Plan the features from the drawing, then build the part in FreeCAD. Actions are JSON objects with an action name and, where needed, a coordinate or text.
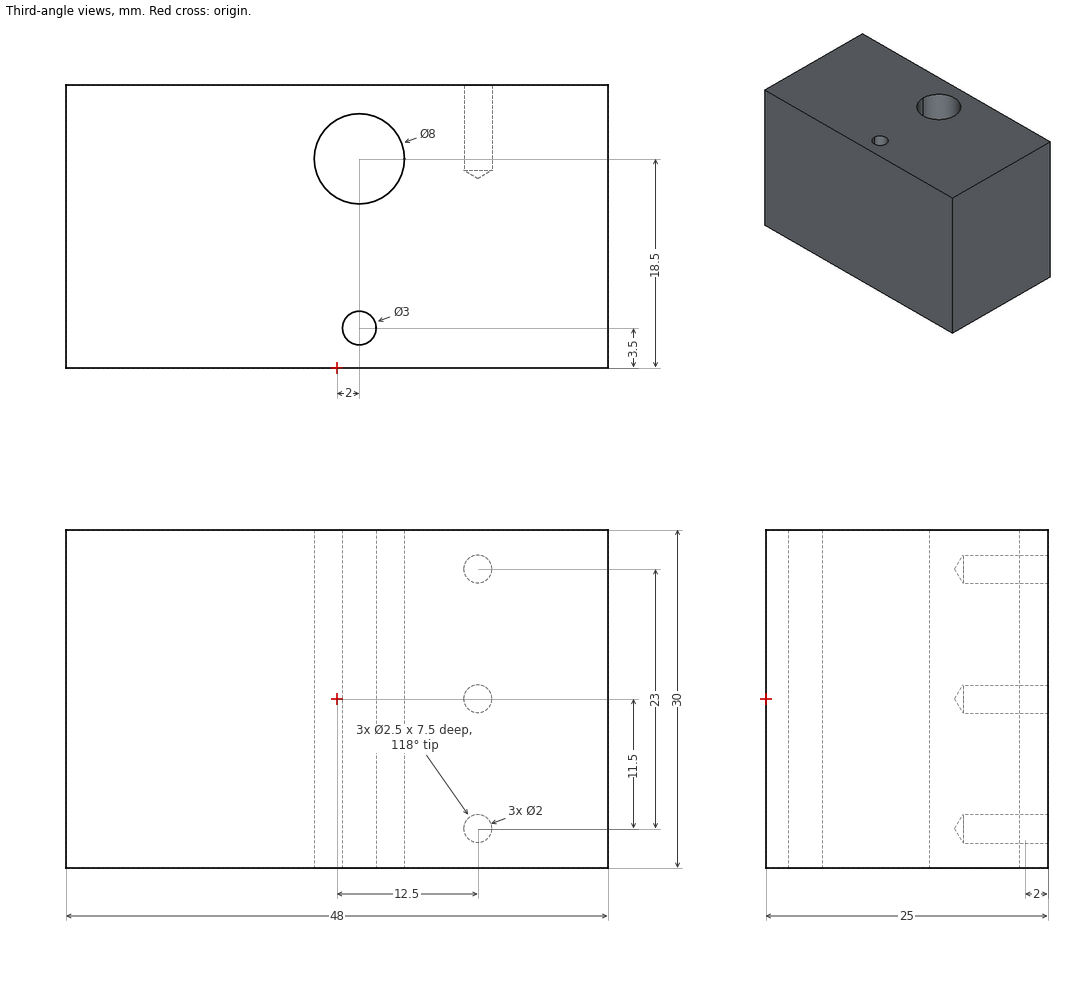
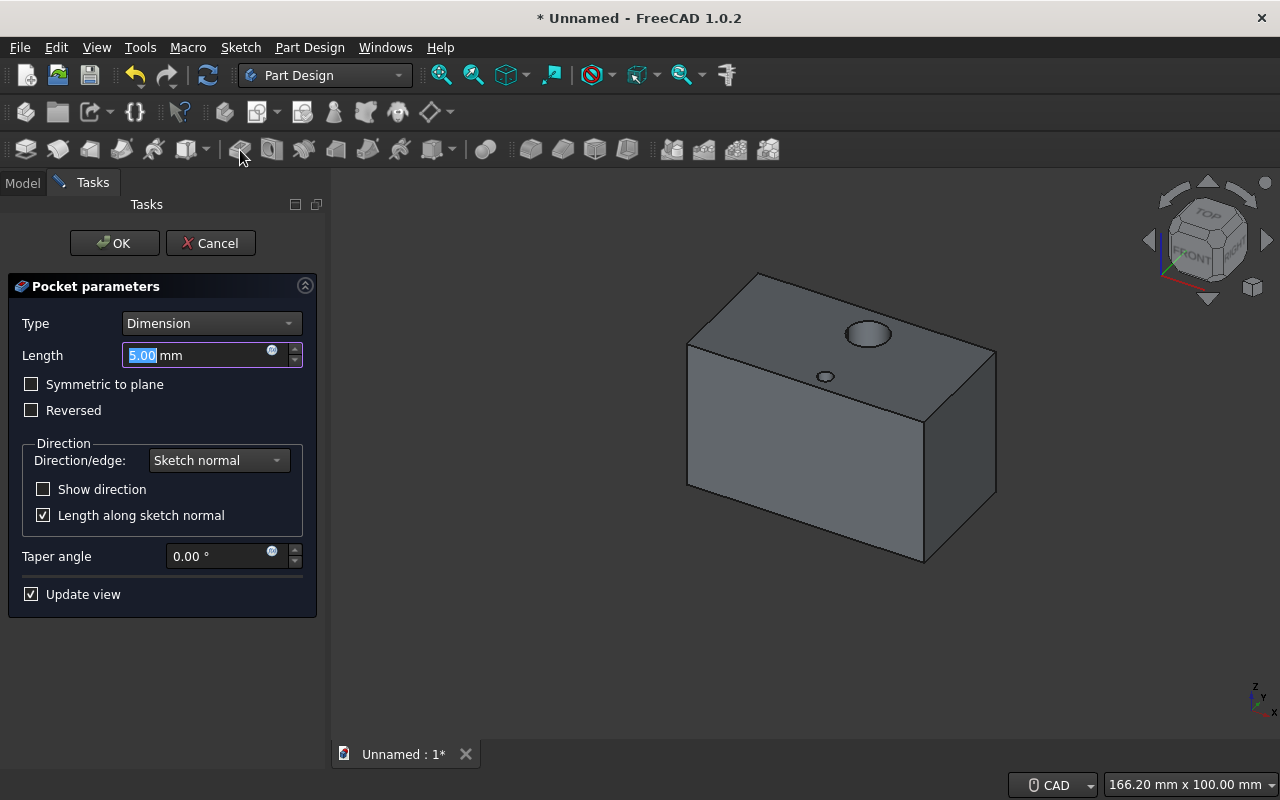
{"action": "left_click", "coordinate": [212, 324]}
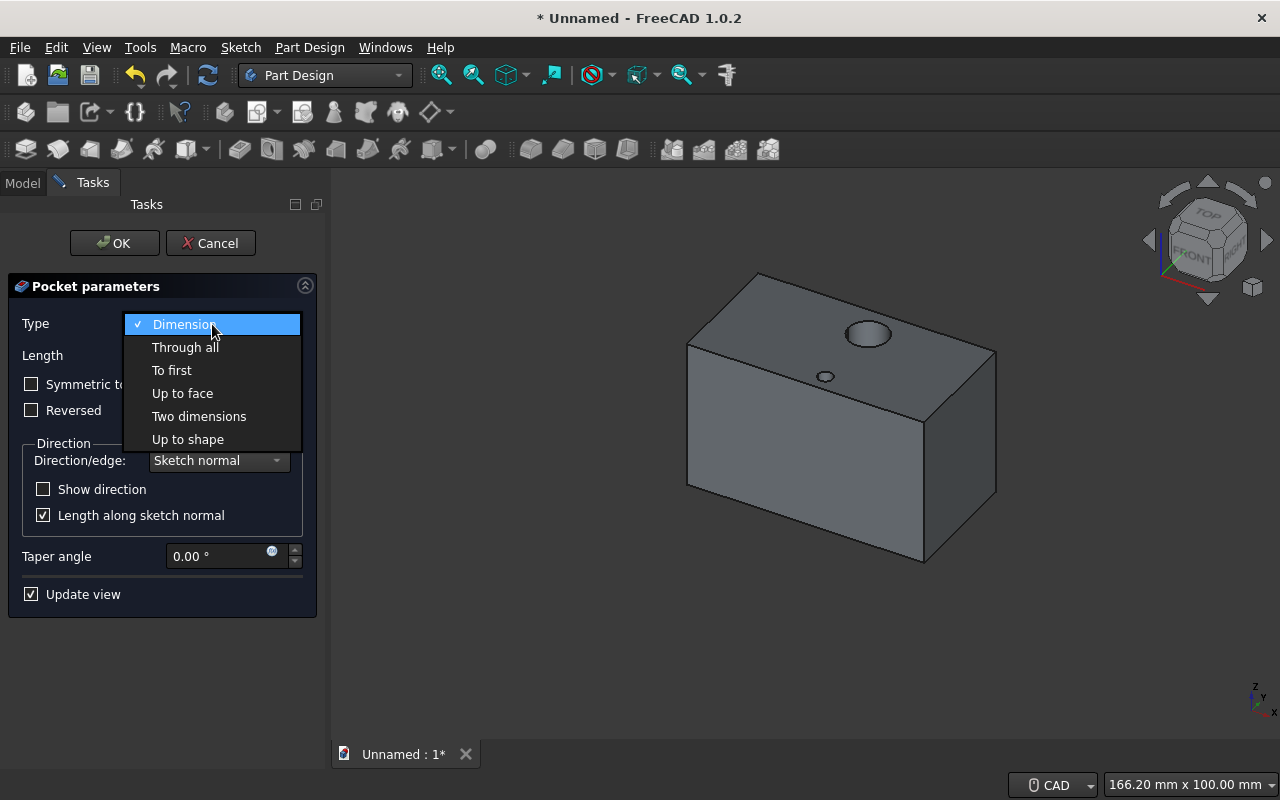
{"action": "left_click", "coordinate": [212, 370]}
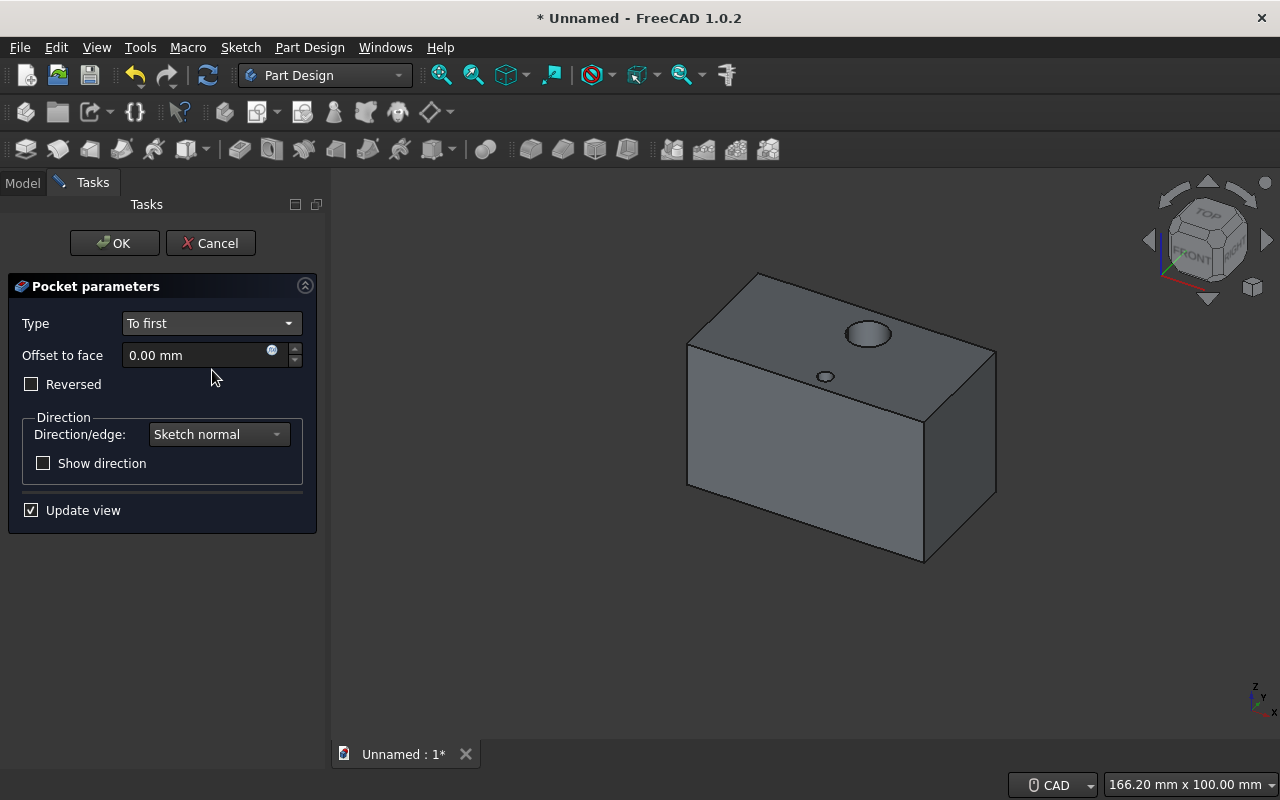
{"action": "left_click", "coordinate": [115, 243]}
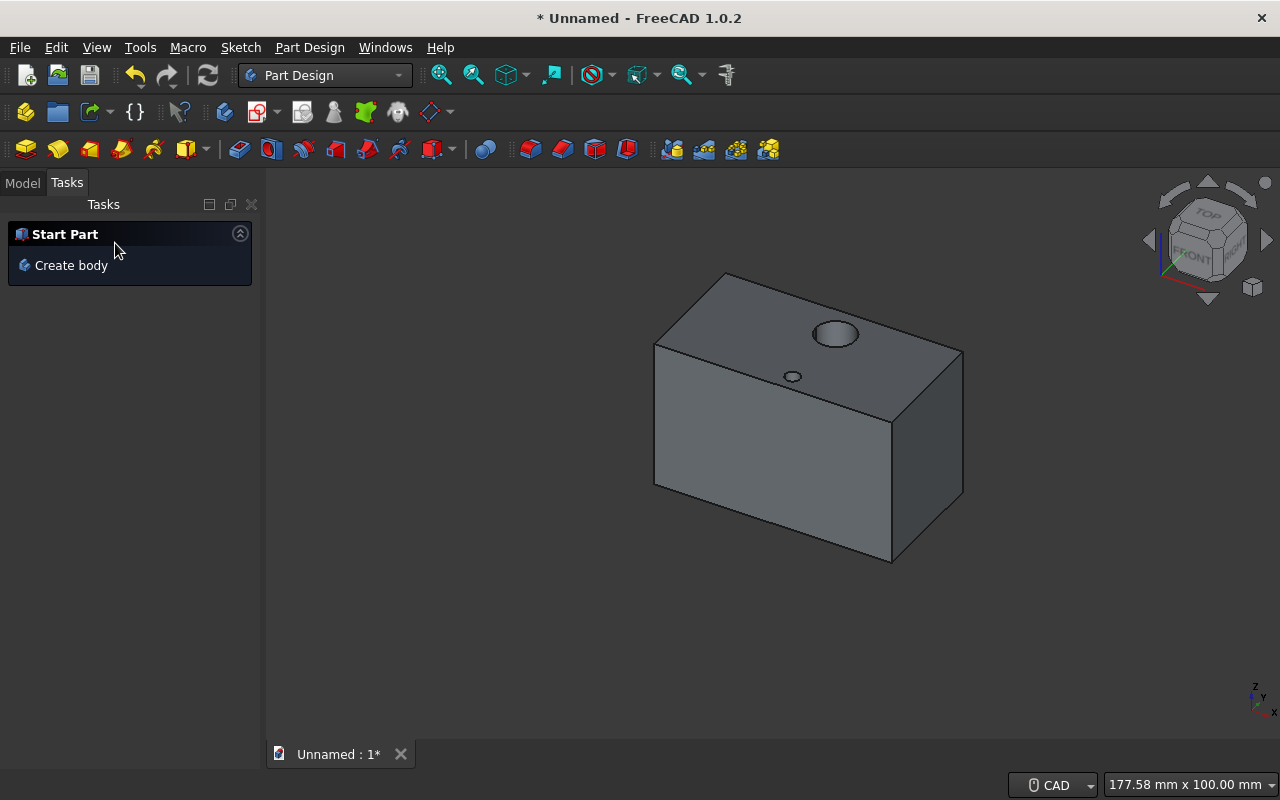
{"action": "key", "text": "4"}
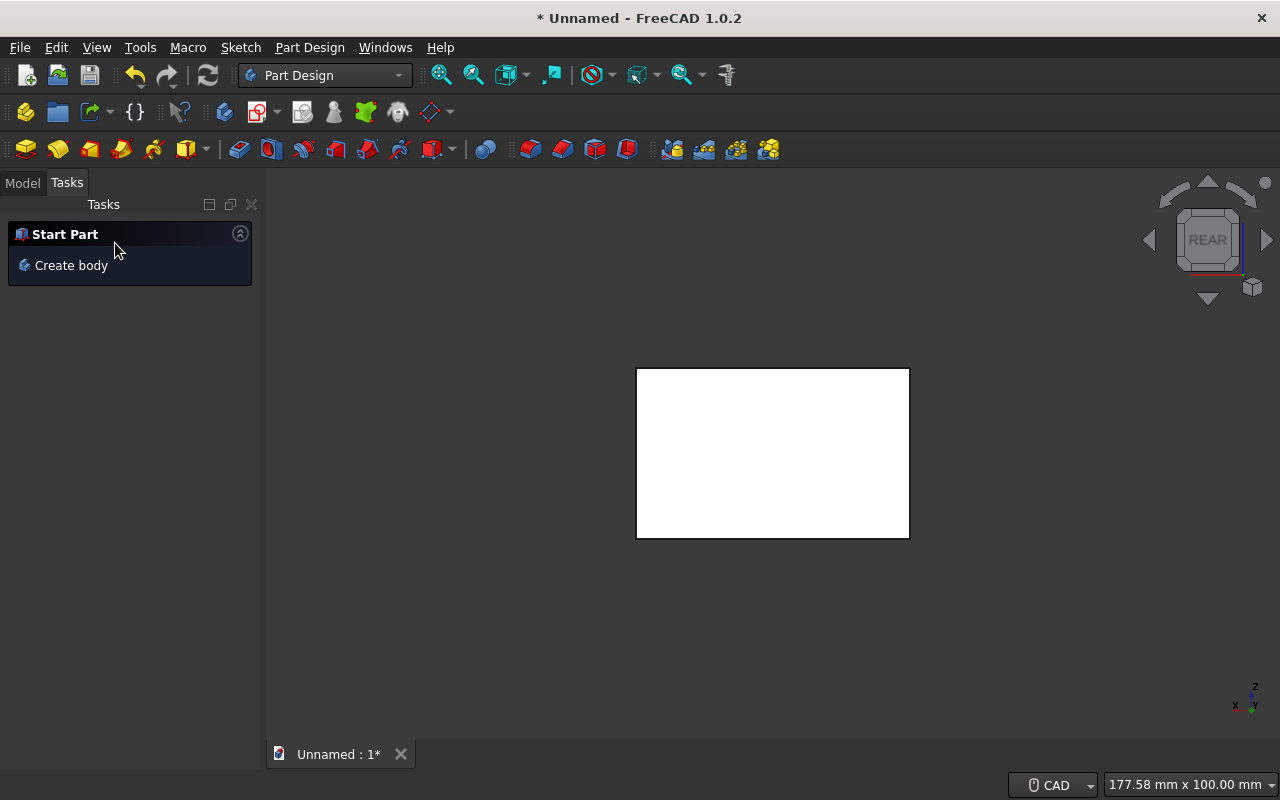
{"action": "key", "text": "v f"}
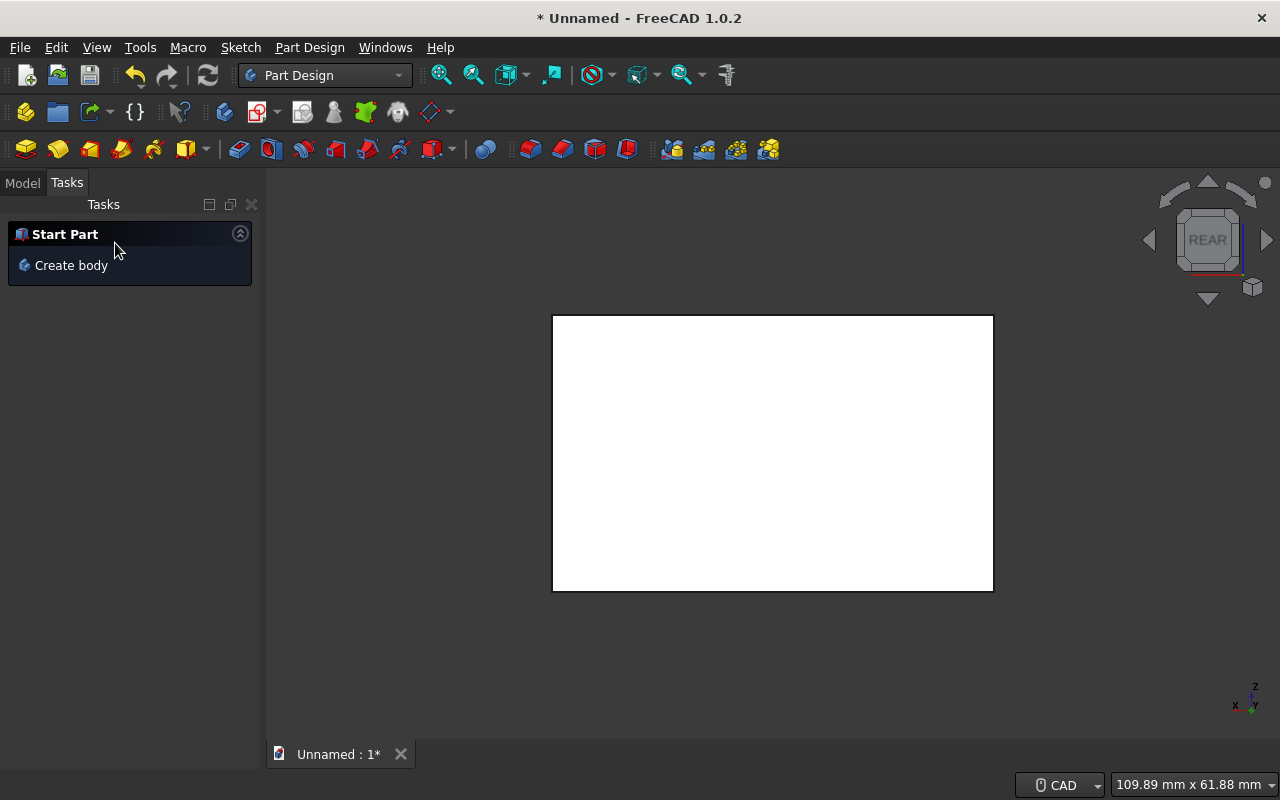
{"action": "left_click", "coordinate": [710, 453]}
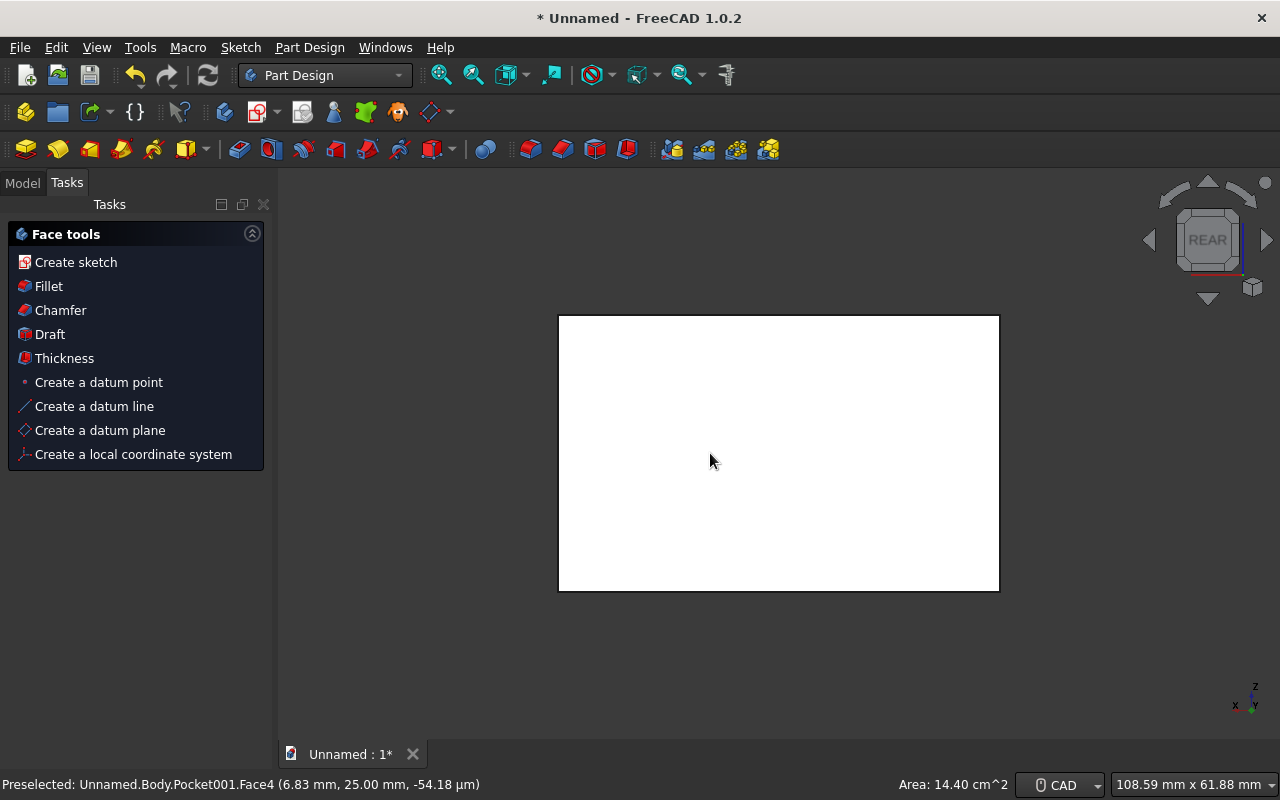
{"action": "left_click", "coordinate": [258, 112]}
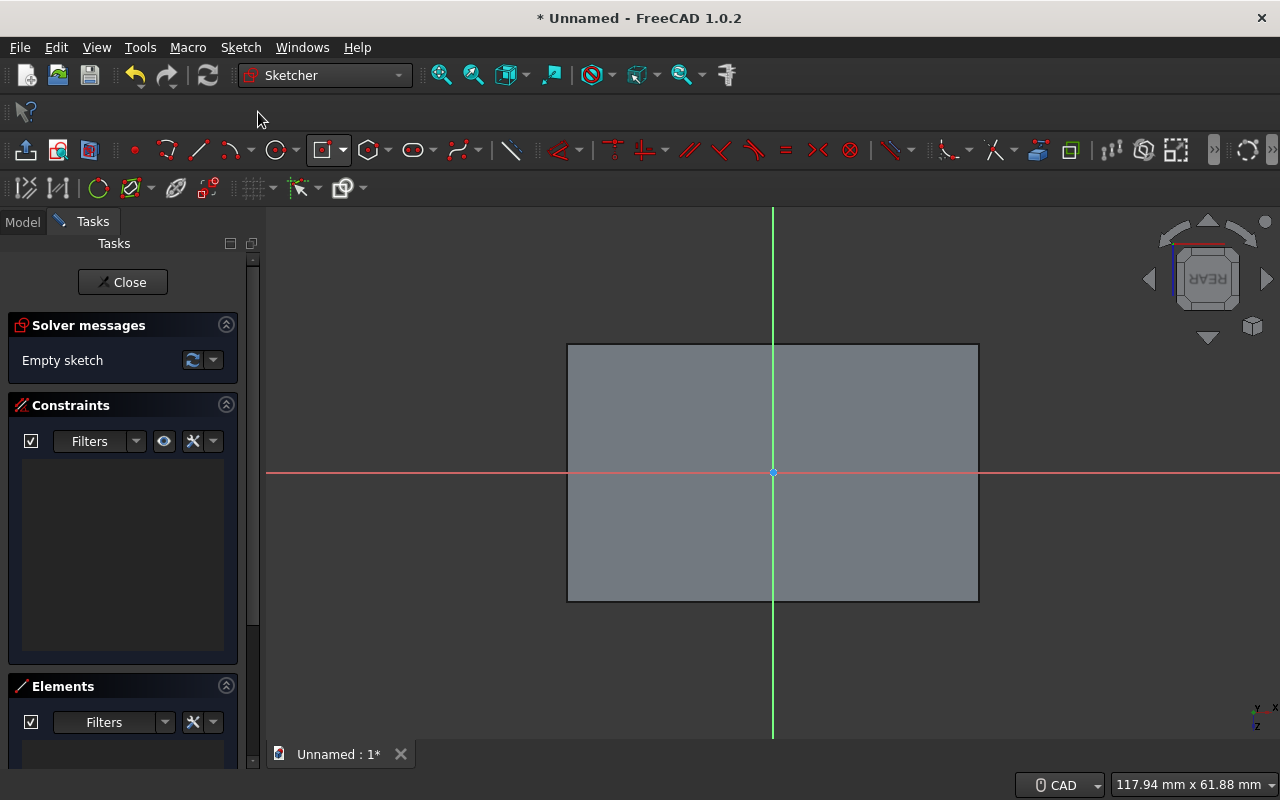
{"action": "scroll", "coordinate": [1088, 473], "scroll_direction": "up", "scroll_amount": 2}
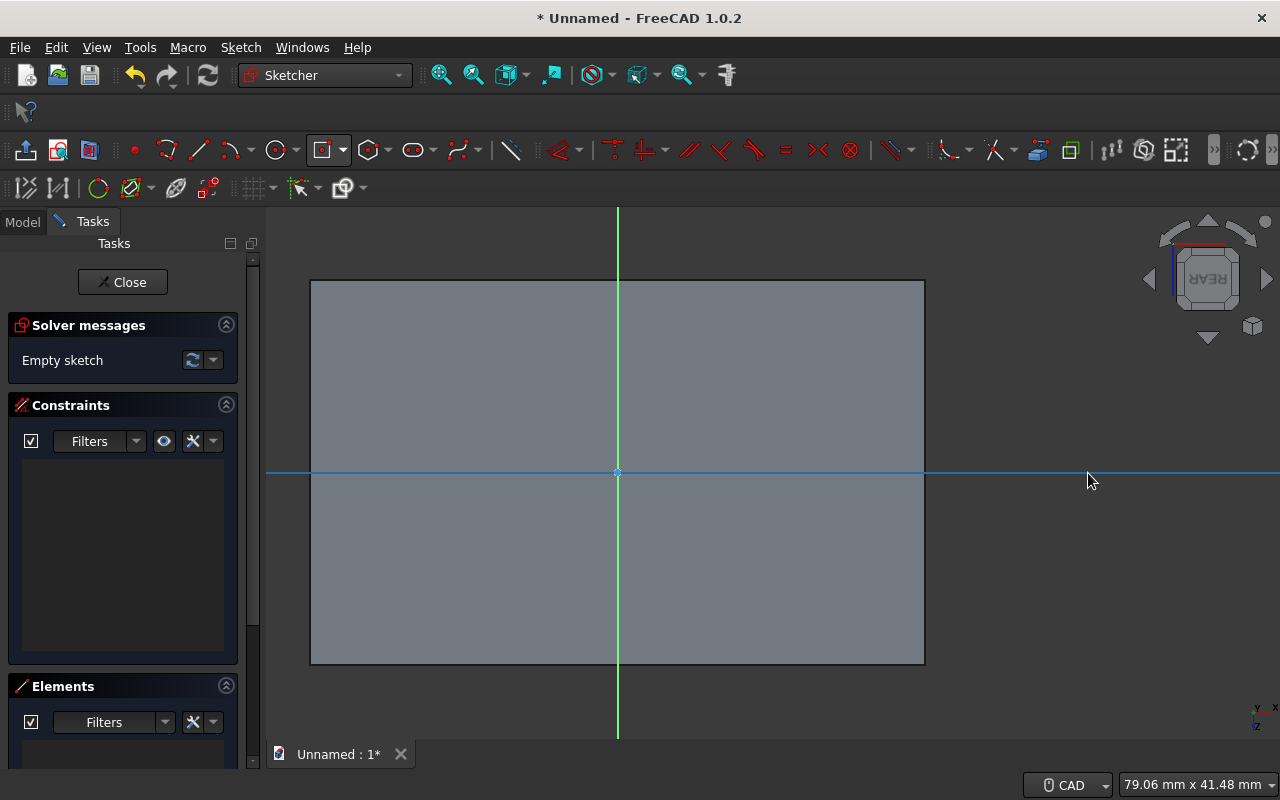
{"action": "key", "text": "g c"}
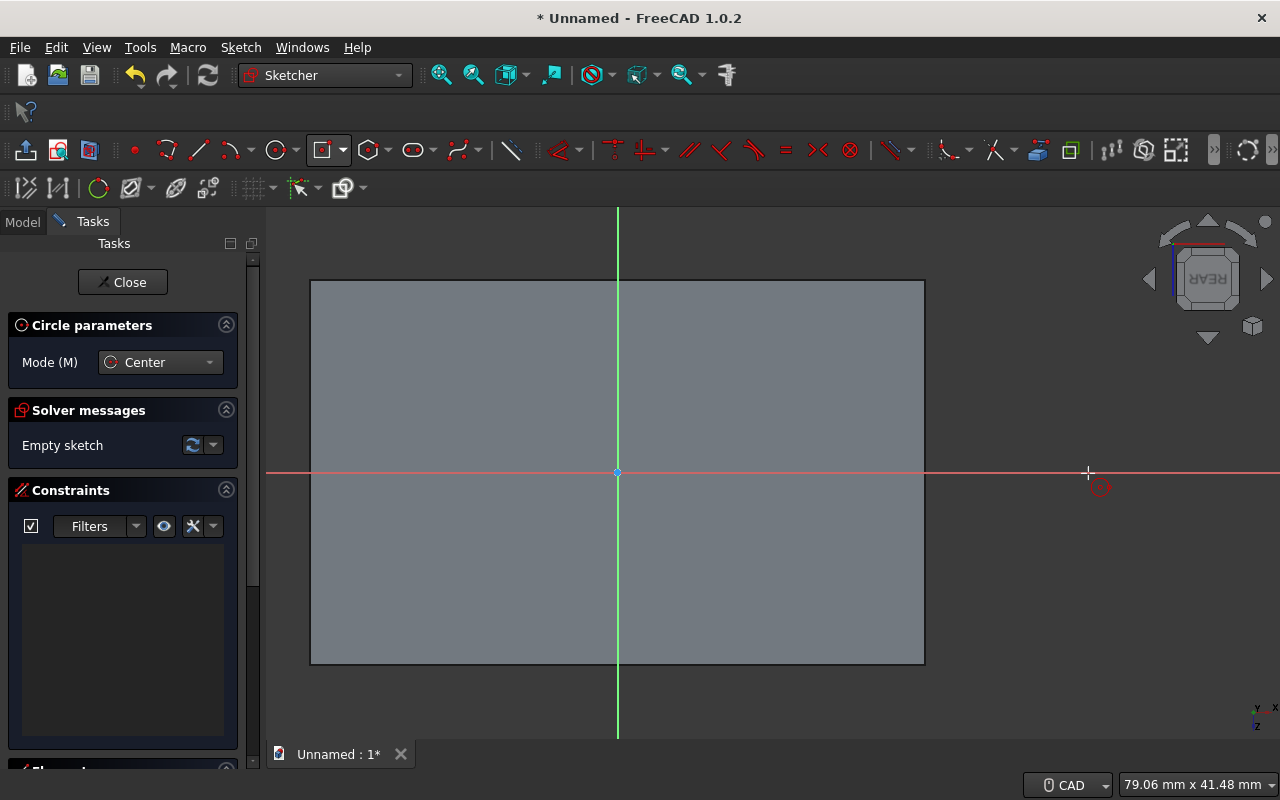
{"action": "scroll", "coordinate": [778, 325], "scroll_direction": "up", "scroll_amount": 3}